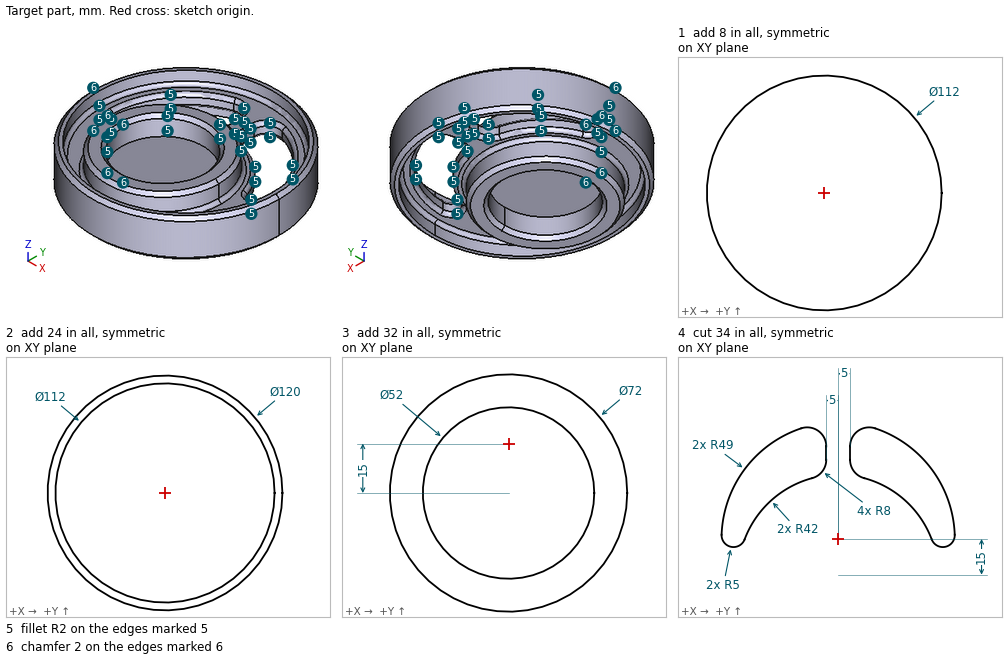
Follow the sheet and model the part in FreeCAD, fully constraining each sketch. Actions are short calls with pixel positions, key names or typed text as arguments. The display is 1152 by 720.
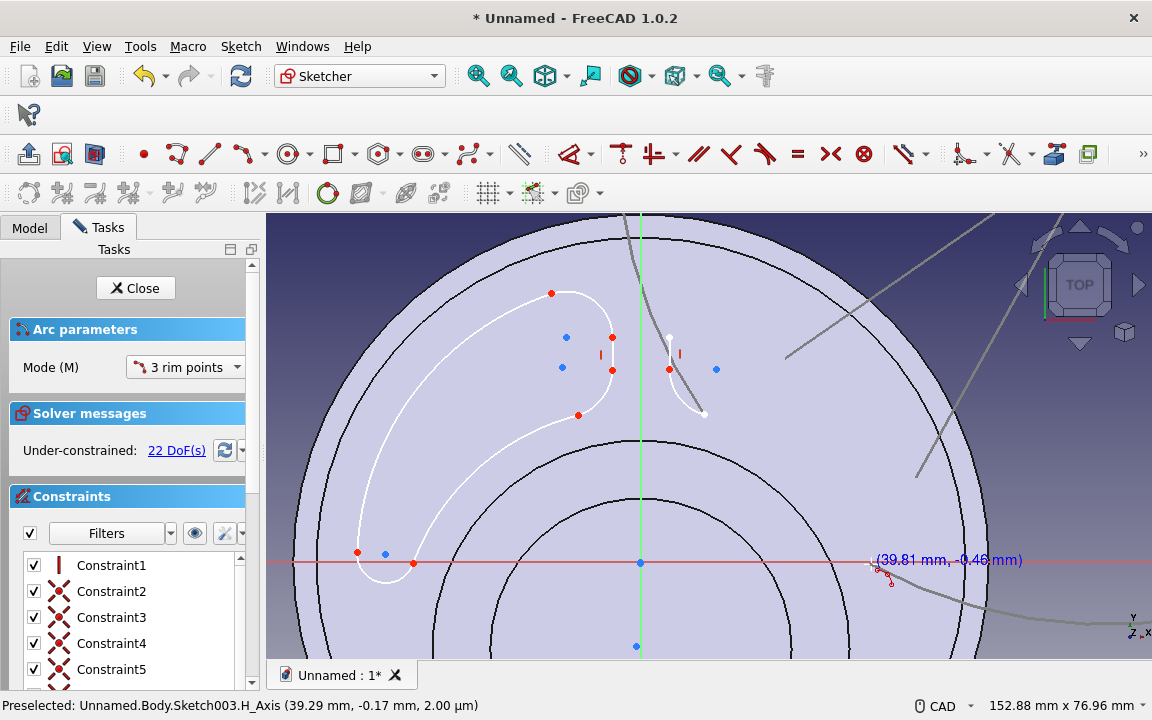
click(804, 469)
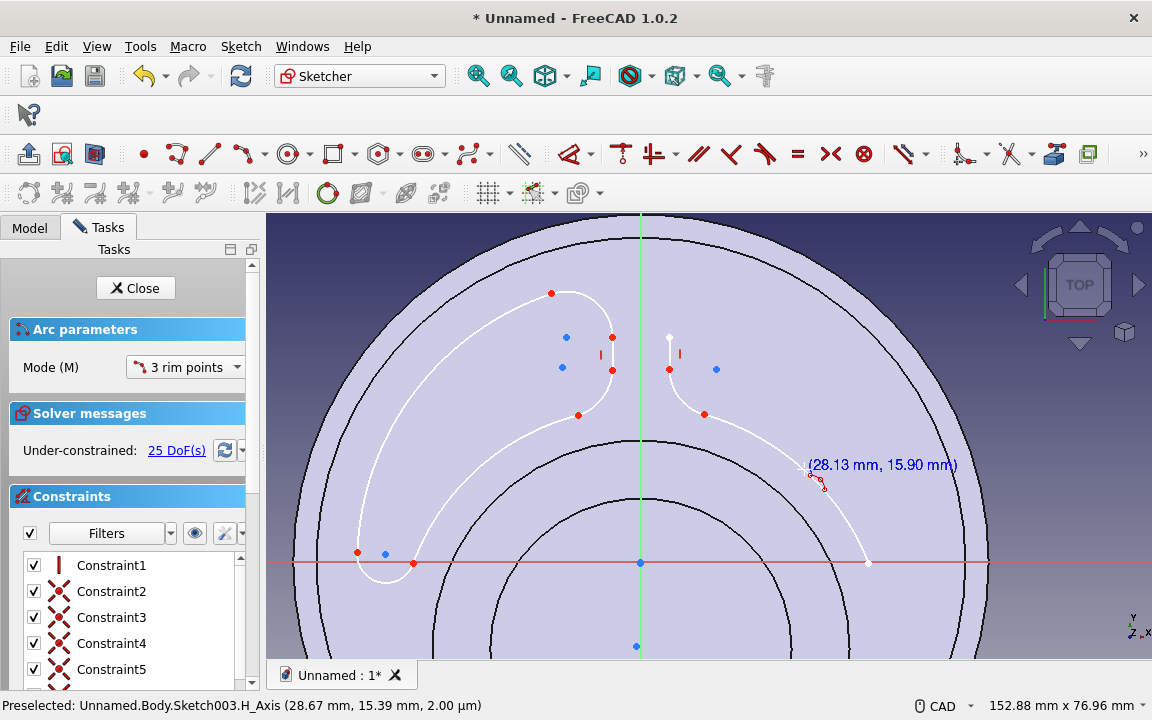
scroll(869, 563, up, 15)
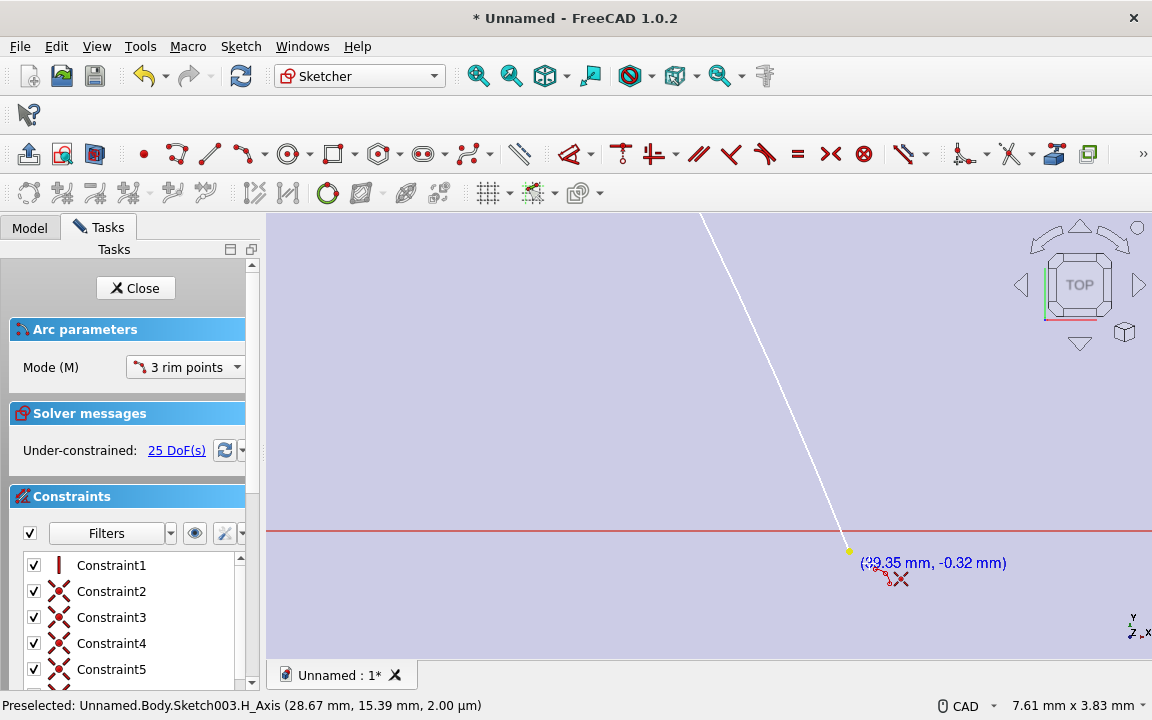
click(849, 551)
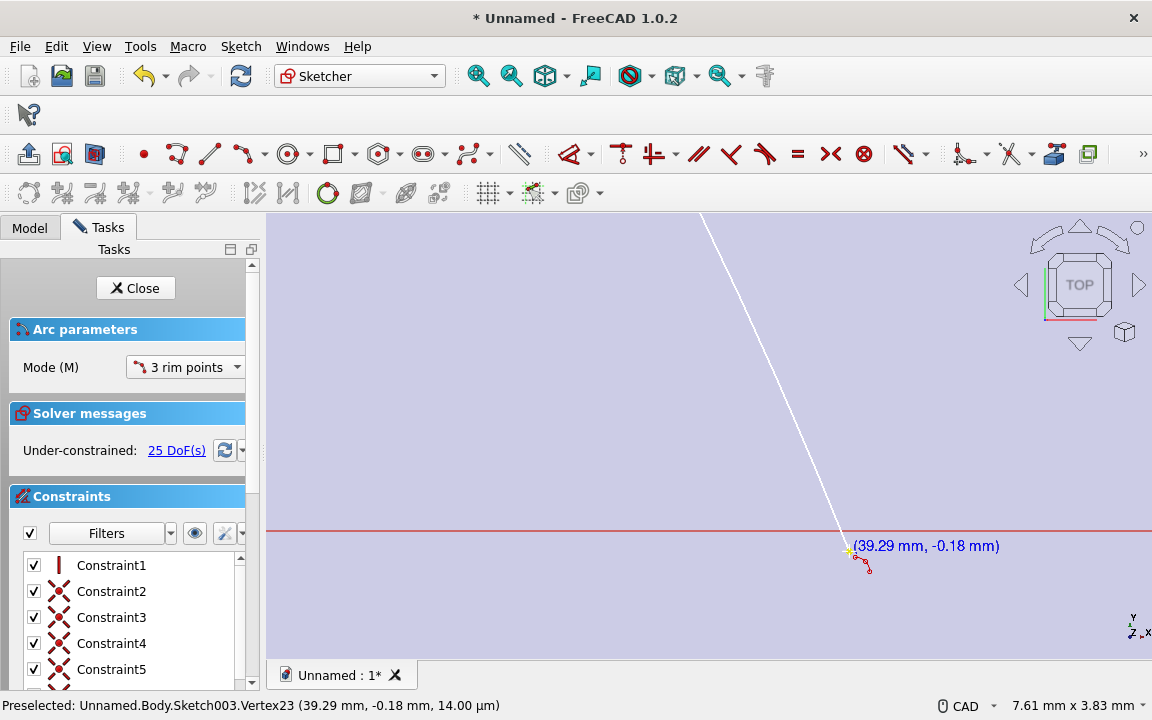
scroll(869, 563, down, 15)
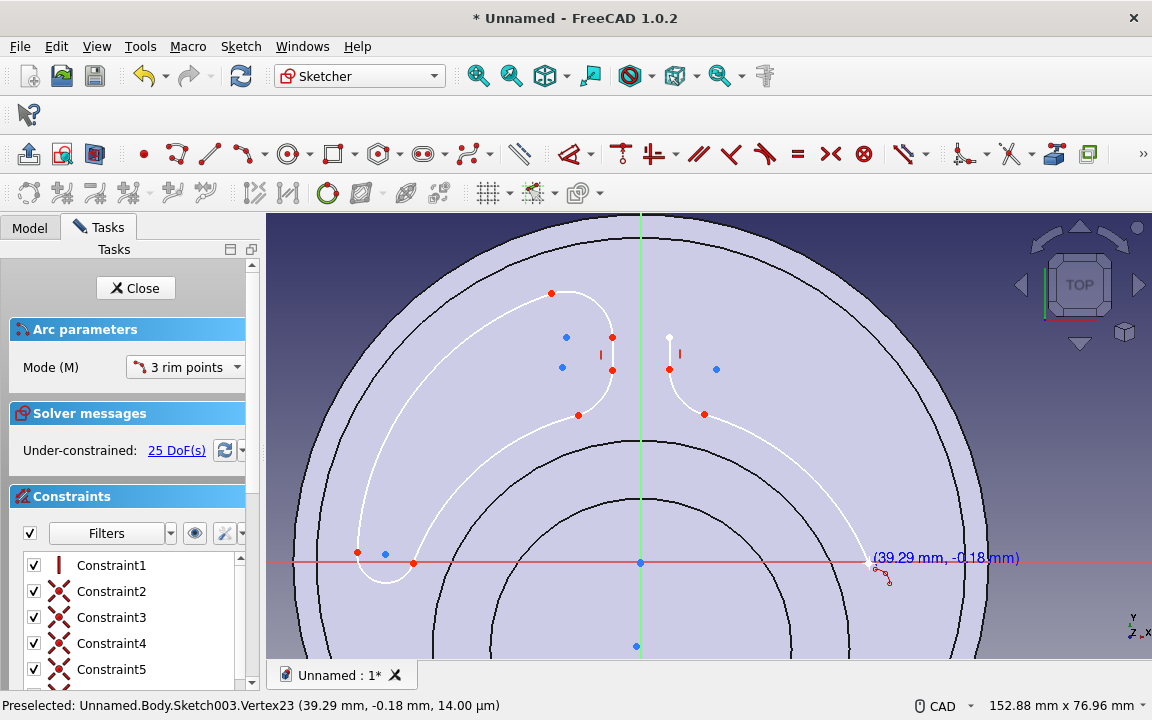
scroll(925, 552, up, 3)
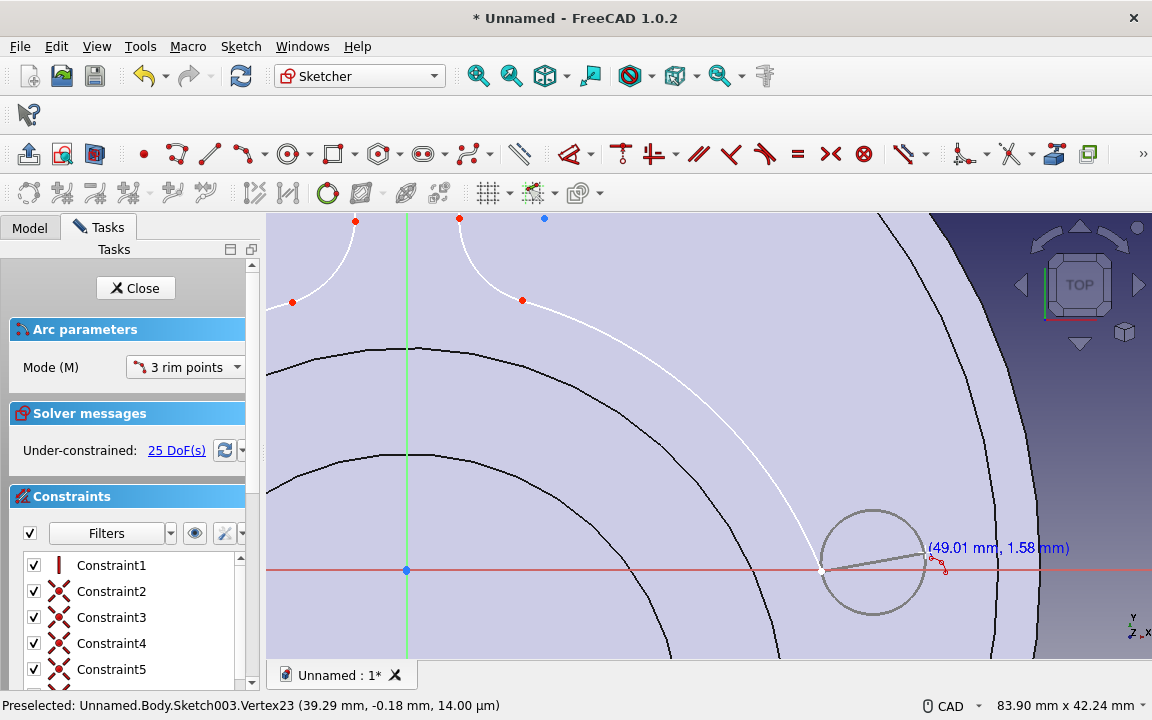
click(924, 551)
click(882, 605)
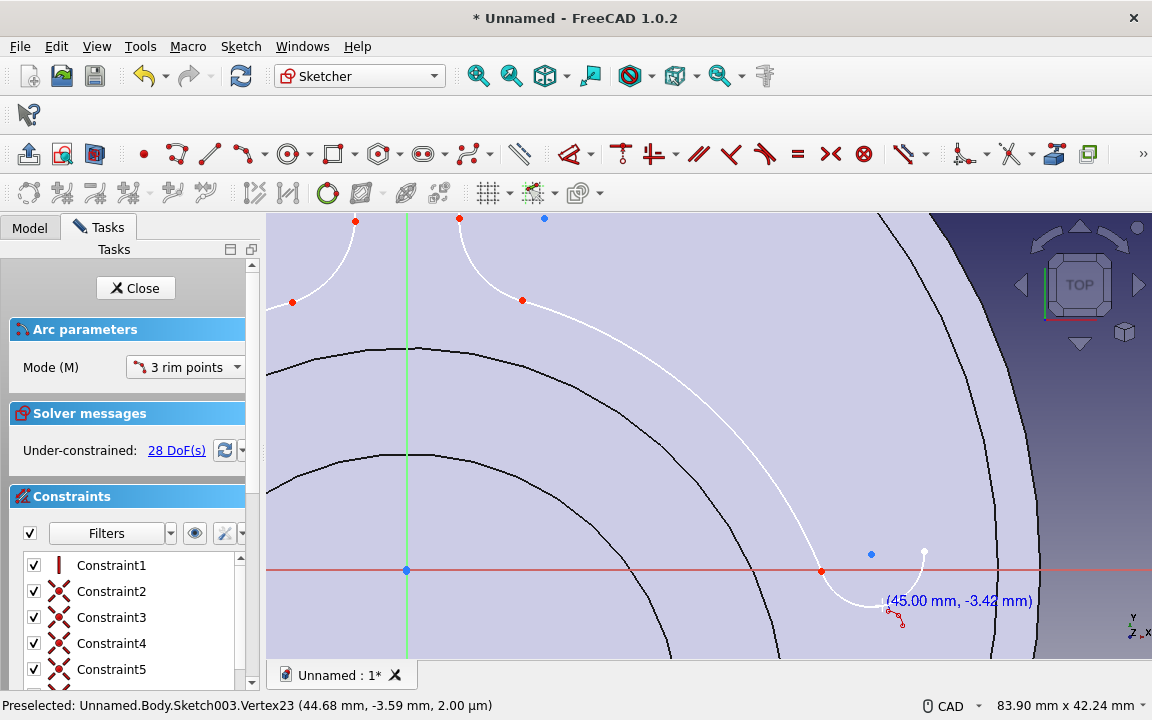
click(924, 552)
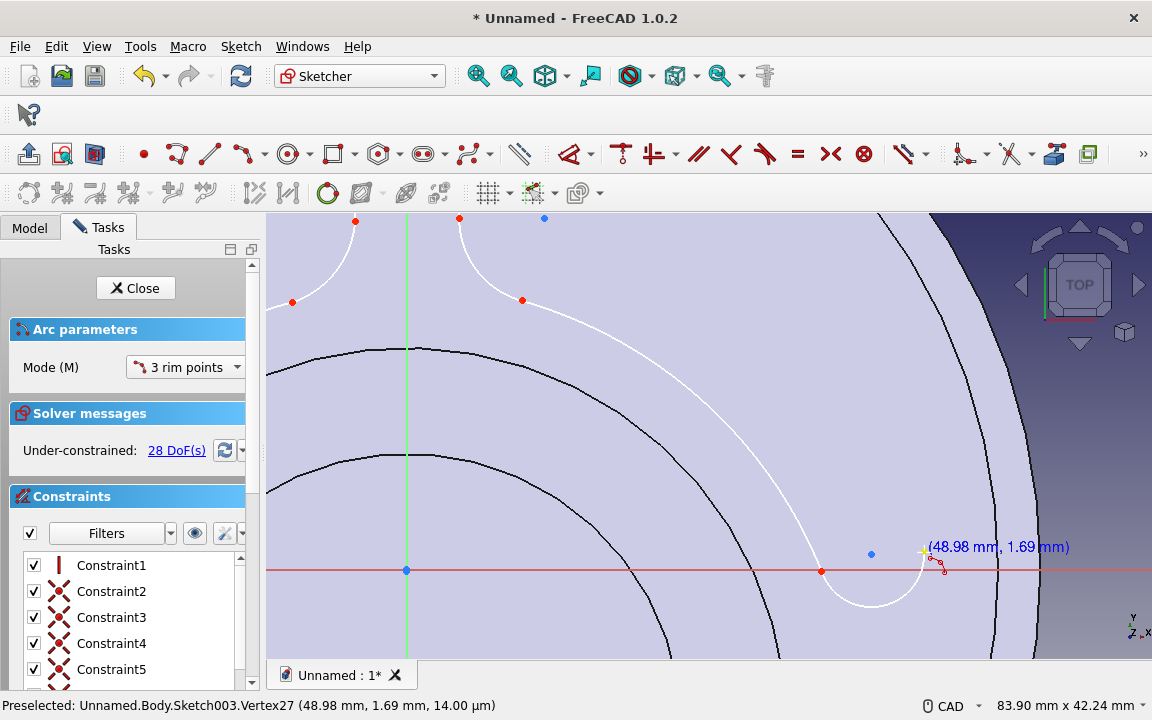
scroll(831, 513, down, 4)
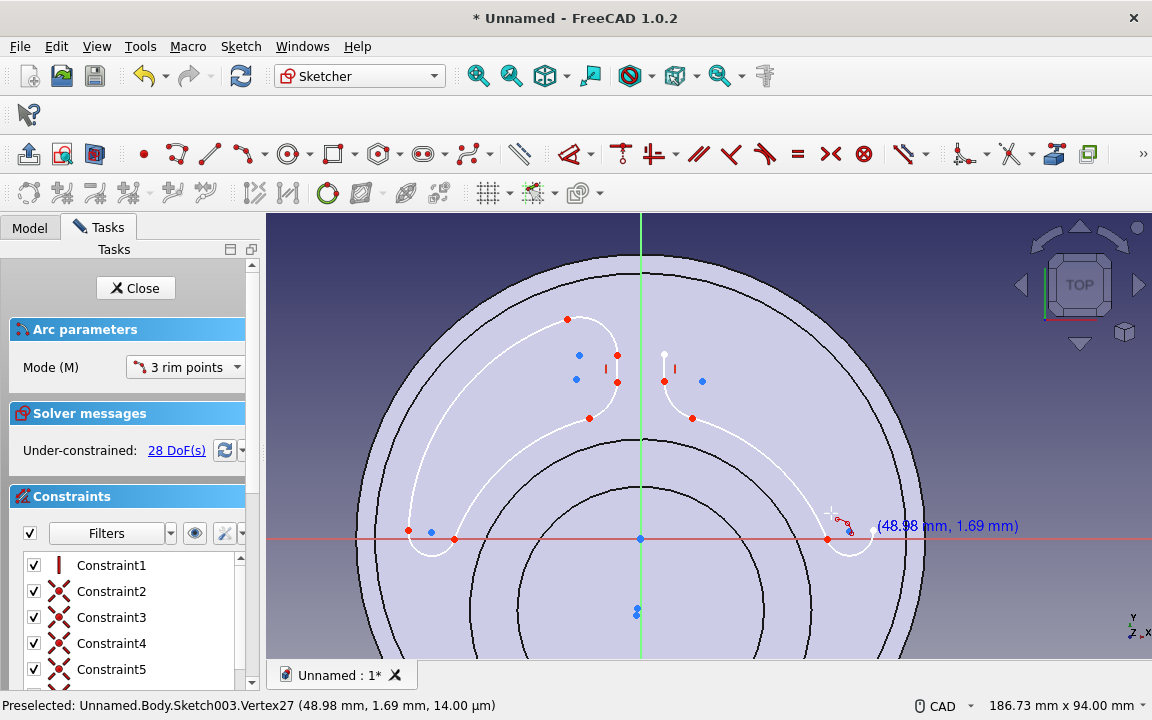
click(714, 318)
click(827, 400)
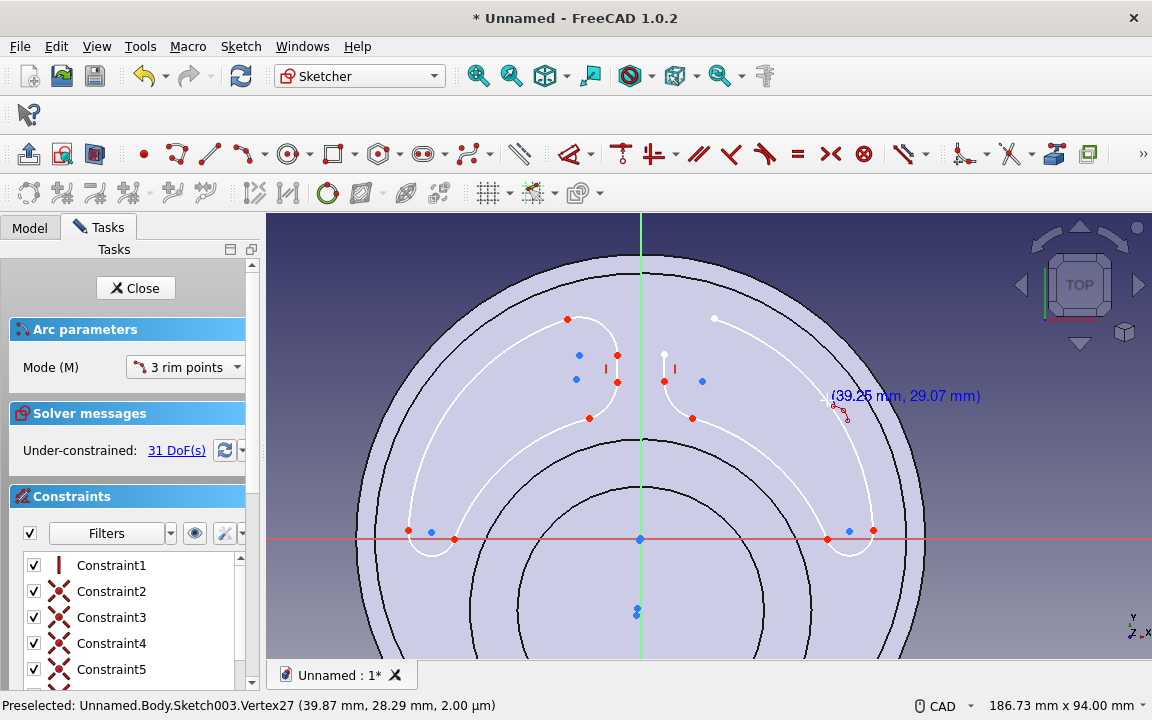
click(714, 319)
click(664, 355)
click(680, 324)
key(Escape)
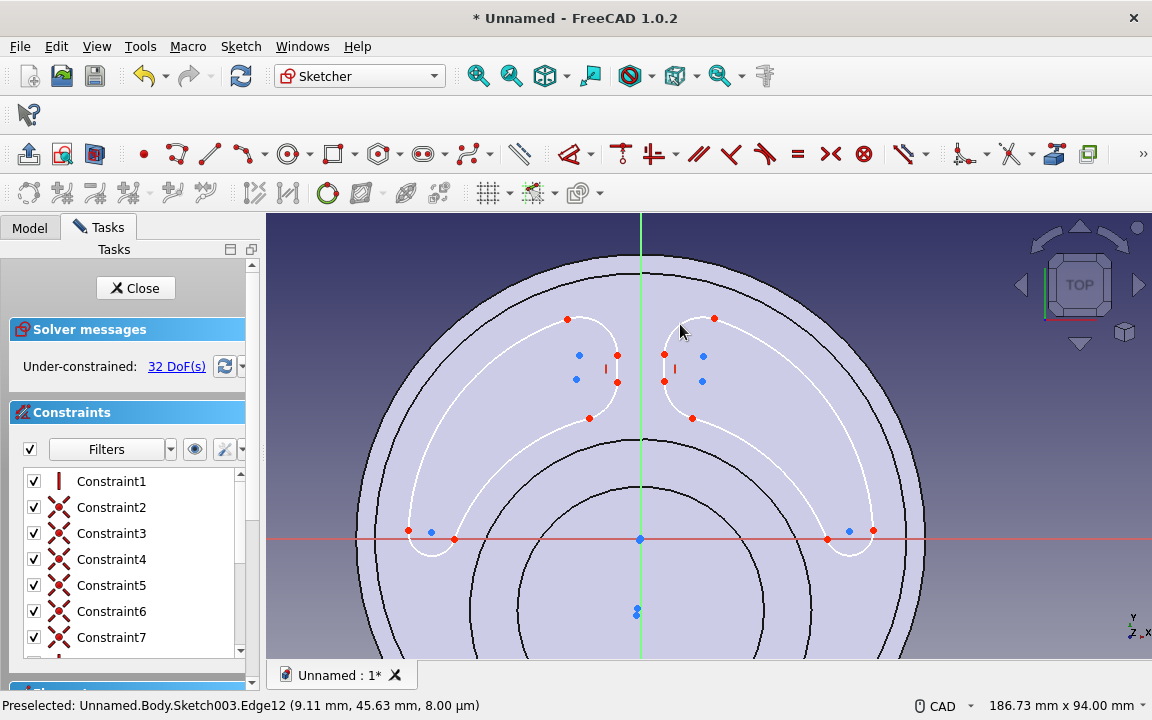
scroll(617, 372, up, 2)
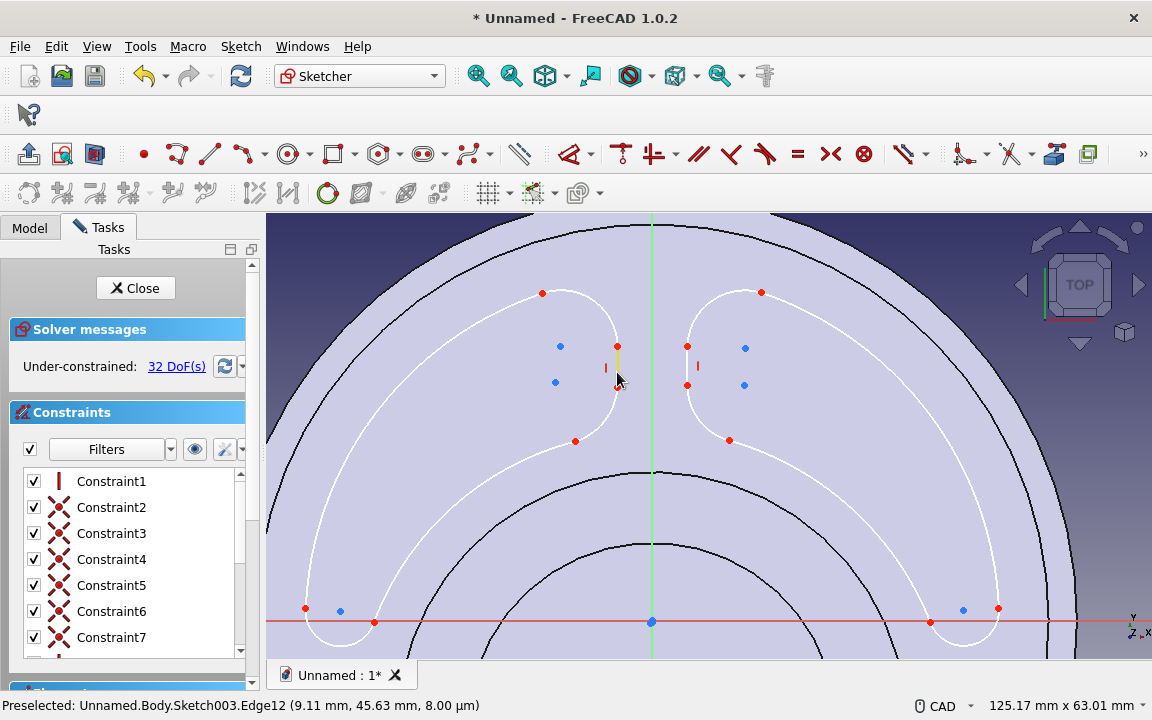
click(618, 371)